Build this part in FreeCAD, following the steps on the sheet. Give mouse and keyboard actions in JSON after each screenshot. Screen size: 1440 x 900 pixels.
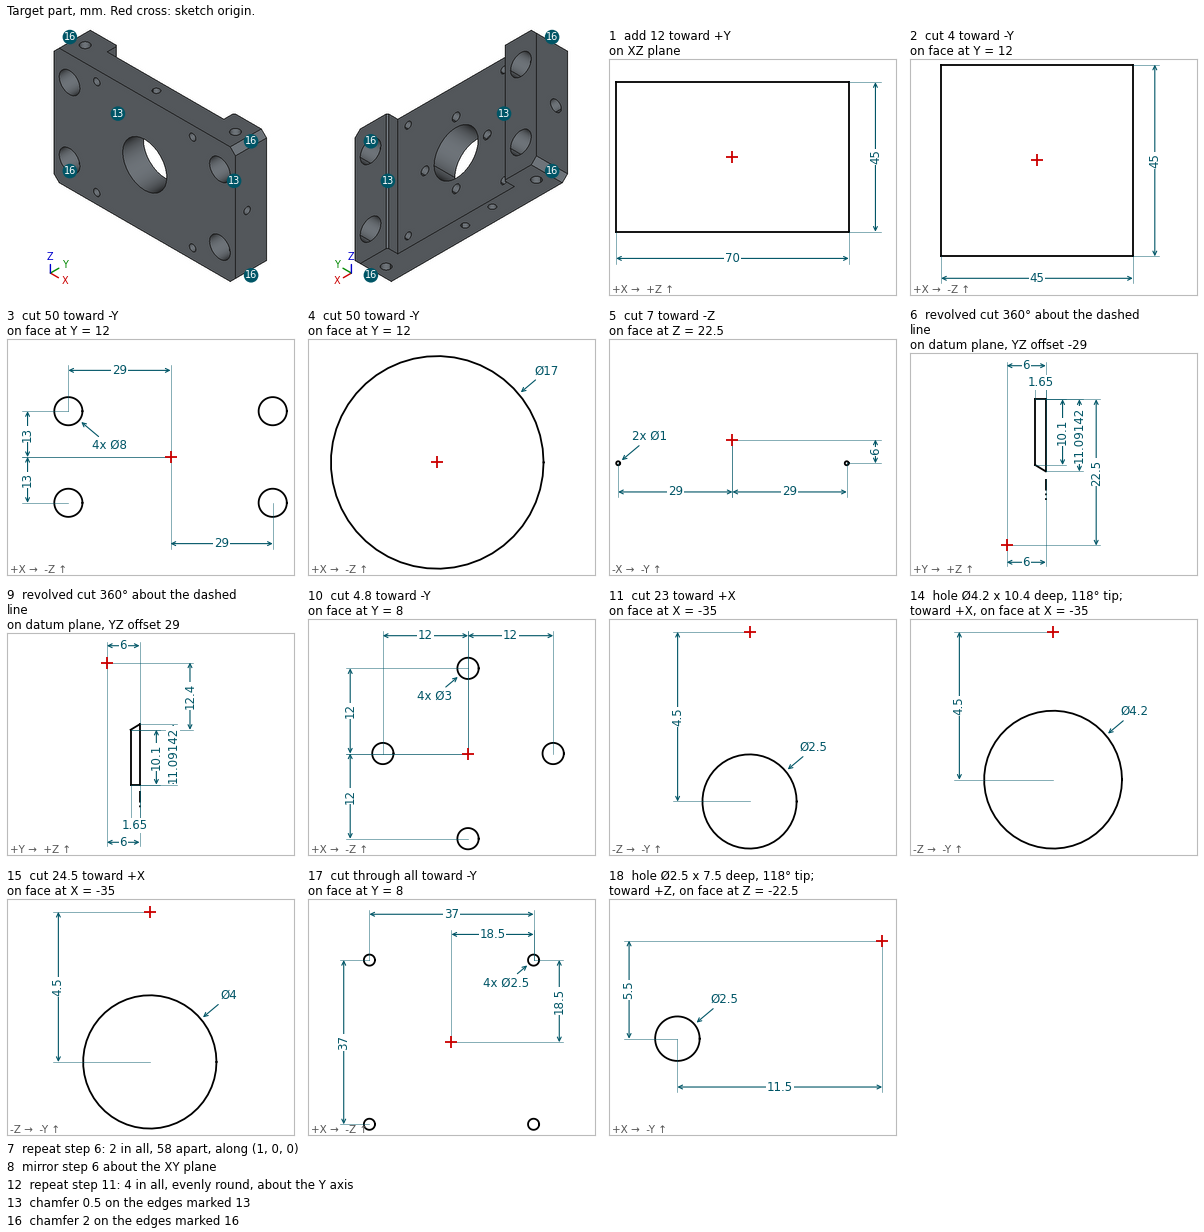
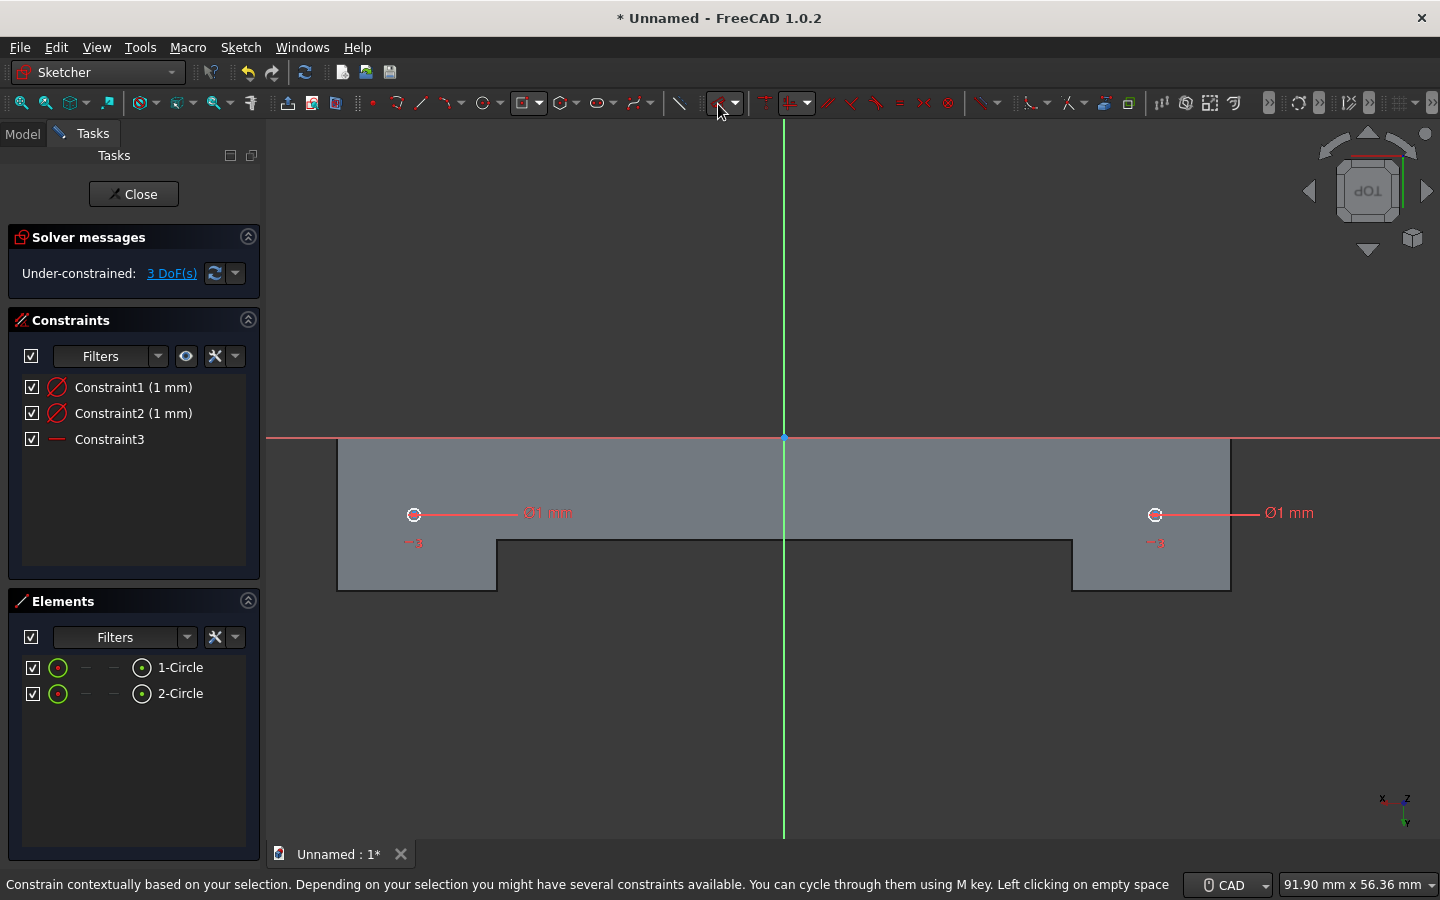
{"action": "left_click", "coordinate": [1155, 515]}
{"action": "left_click", "coordinate": [1189, 476]}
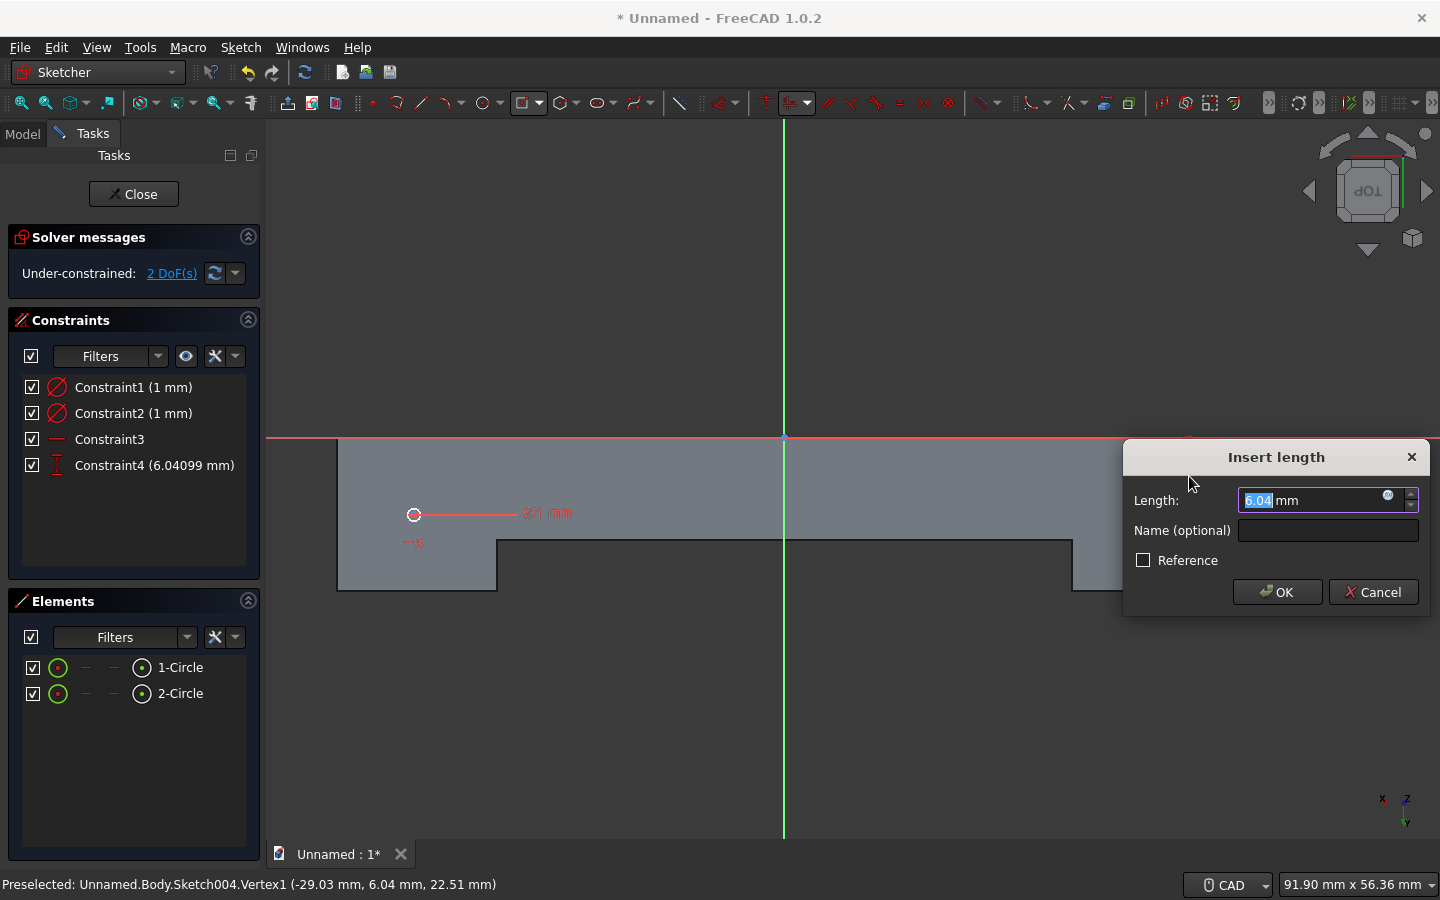
{"action": "type", "text": "6"}
{"action": "key", "text": "Return"}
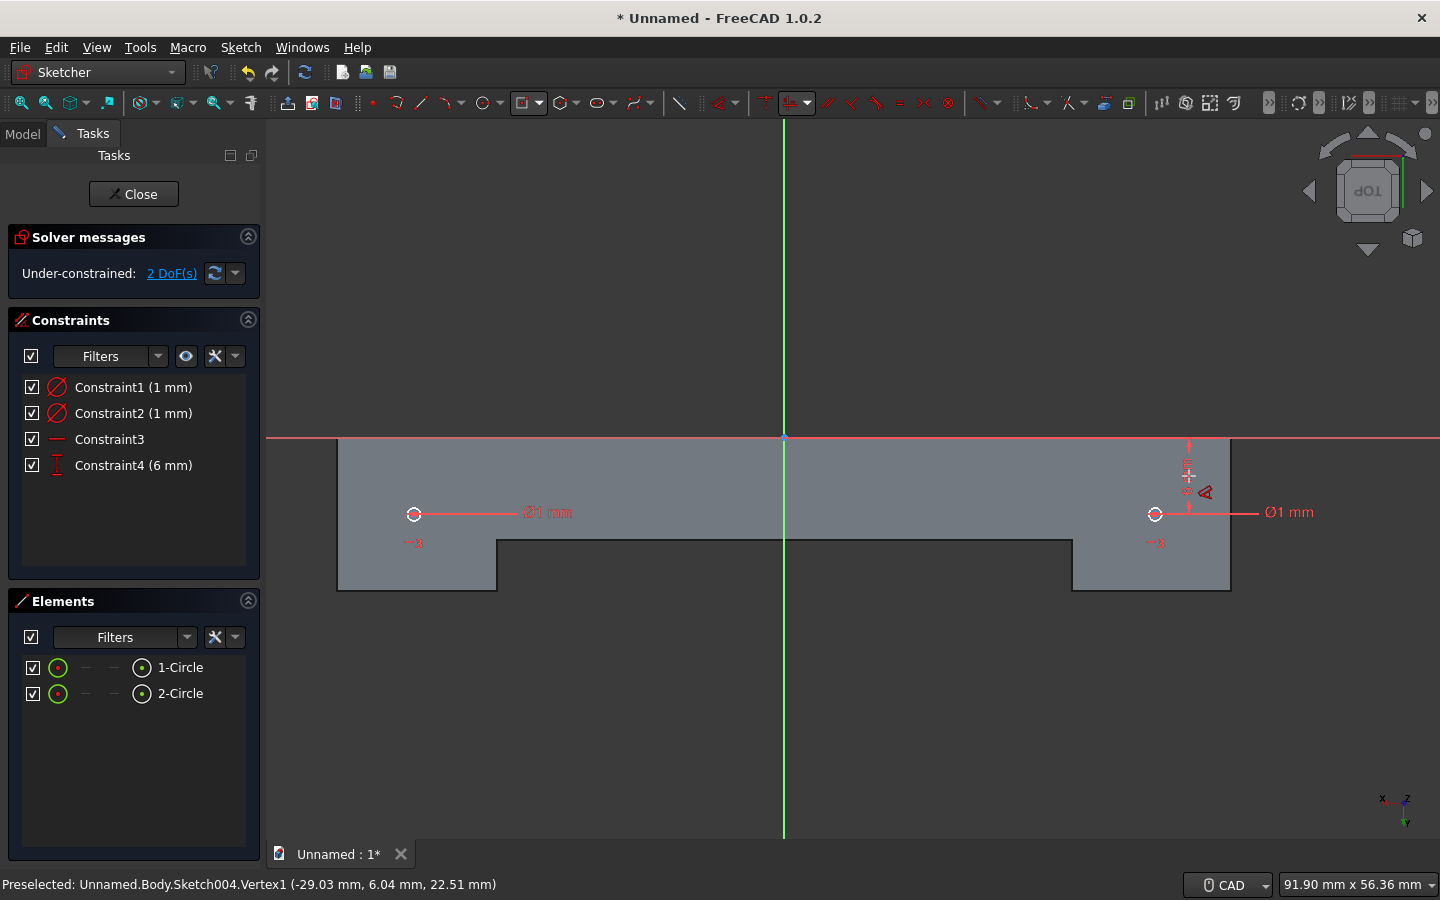
{"action": "left_click", "coordinate": [1155, 514]}
{"action": "left_click", "coordinate": [970, 404]}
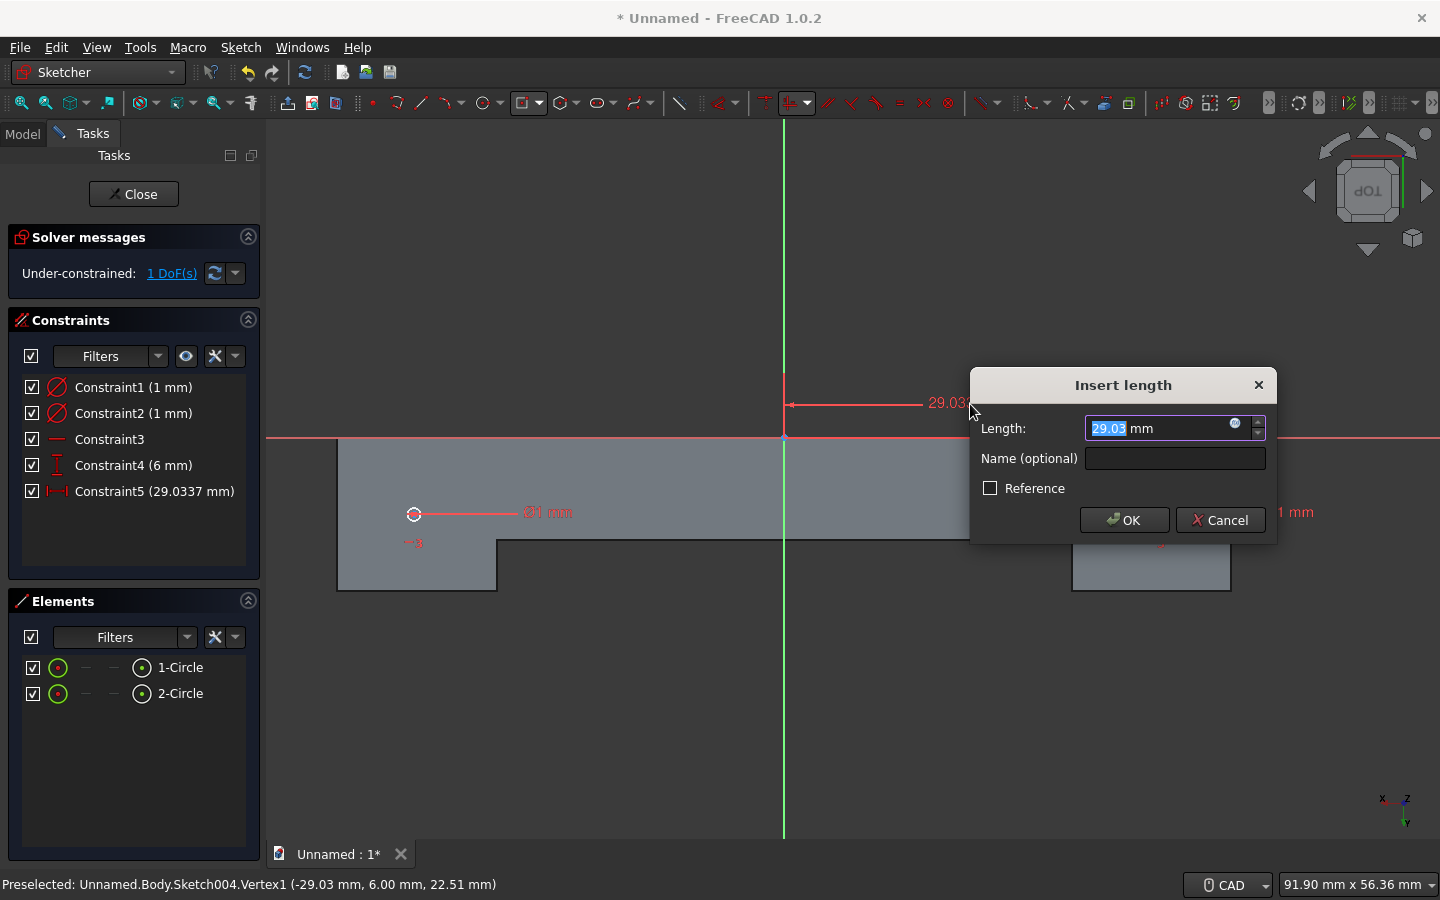
{"action": "type", "text": "29"}
{"action": "key", "text": "Return"}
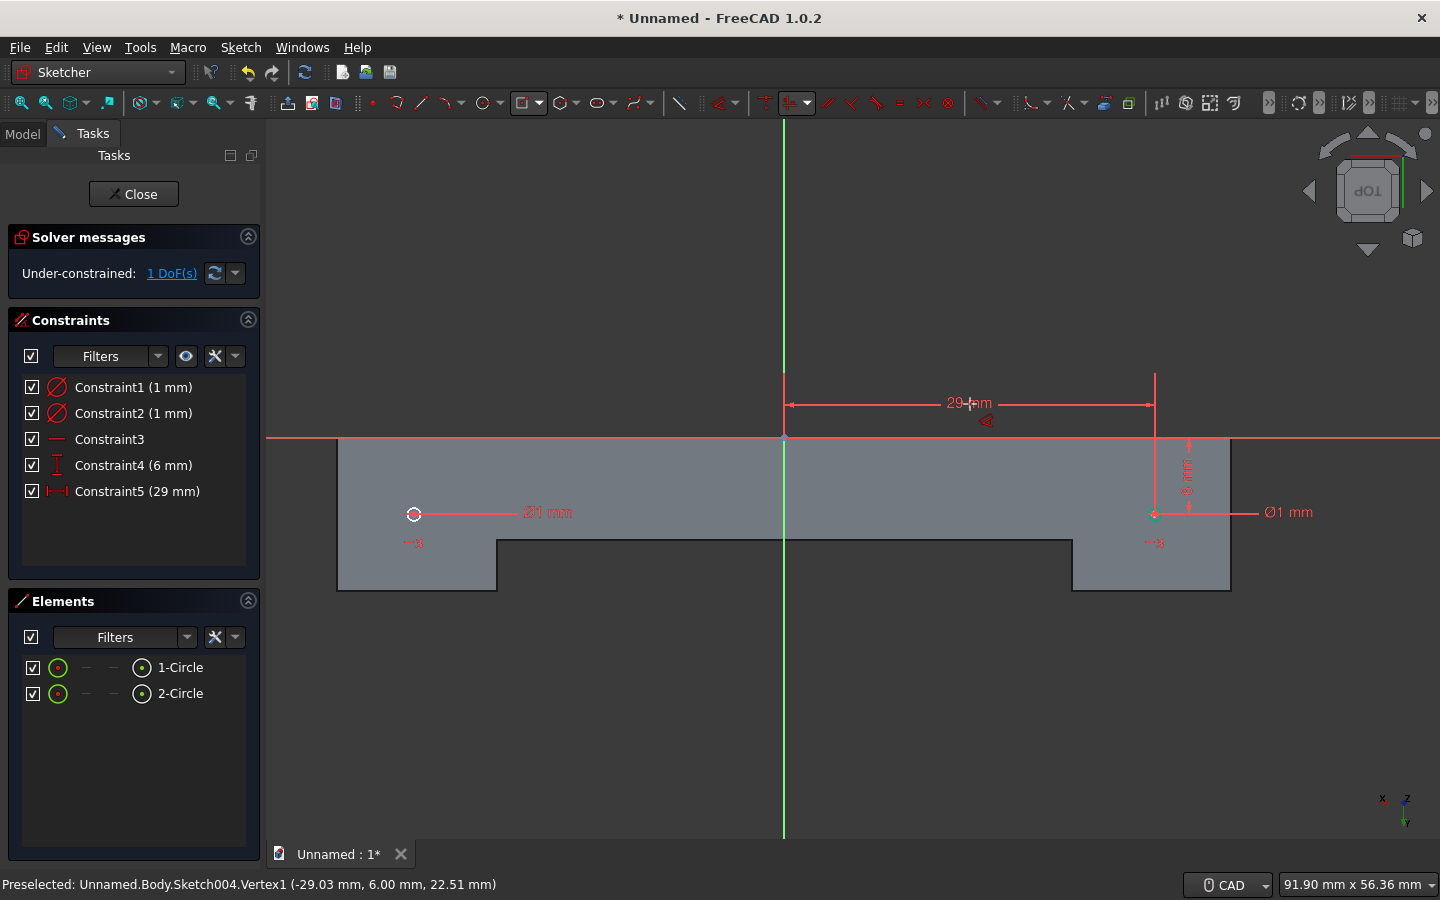
{"action": "left_click", "coordinate": [414, 514]}
{"action": "left_click", "coordinate": [599, 404]}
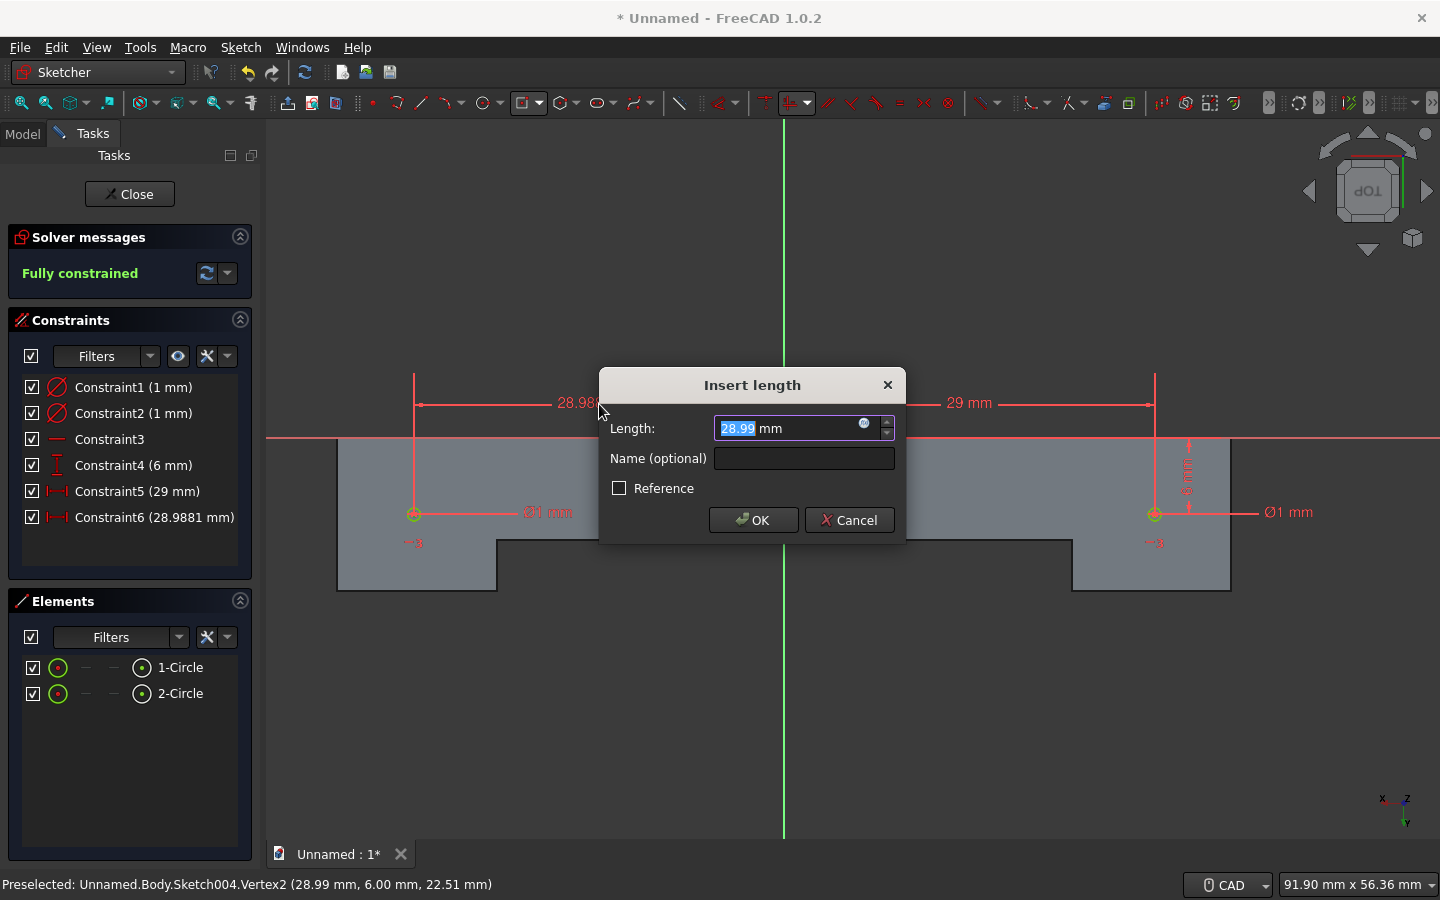
{"action": "type", "text": "29"}
{"action": "key", "text": "Return"}
{"action": "key", "text": "Escape"}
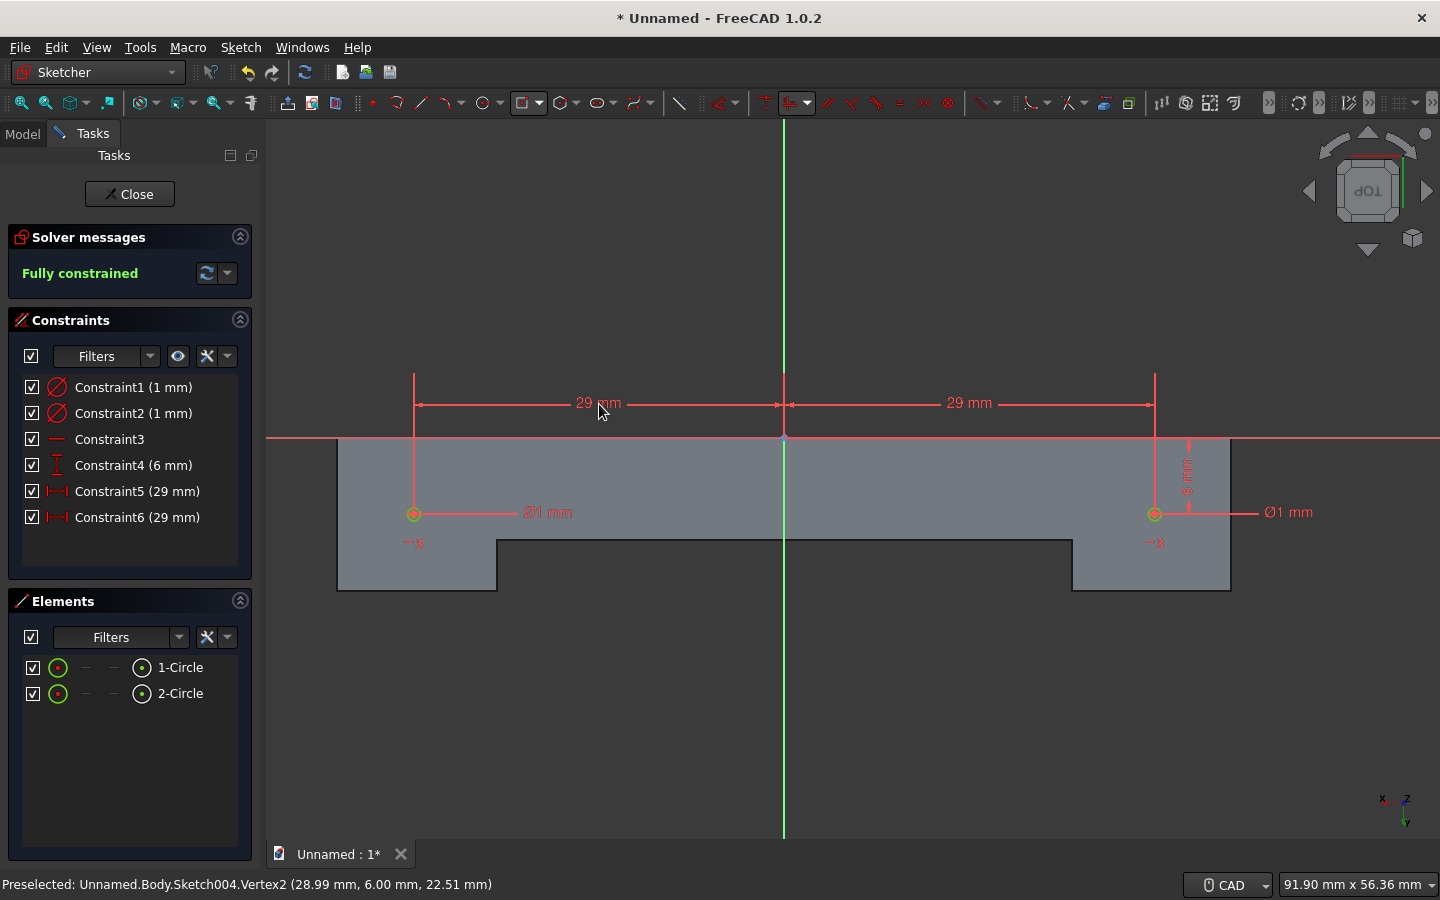
{"action": "left_click", "coordinate": [130, 194]}